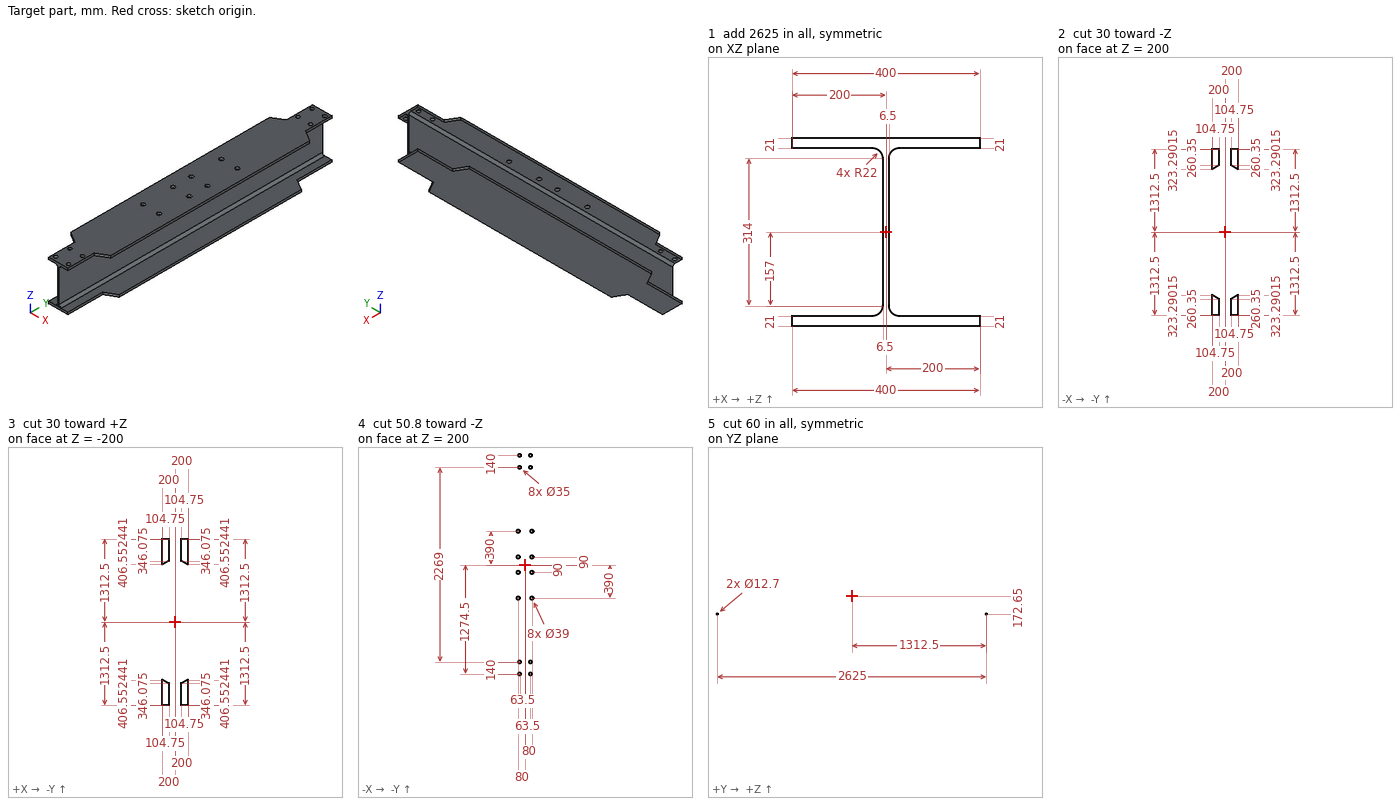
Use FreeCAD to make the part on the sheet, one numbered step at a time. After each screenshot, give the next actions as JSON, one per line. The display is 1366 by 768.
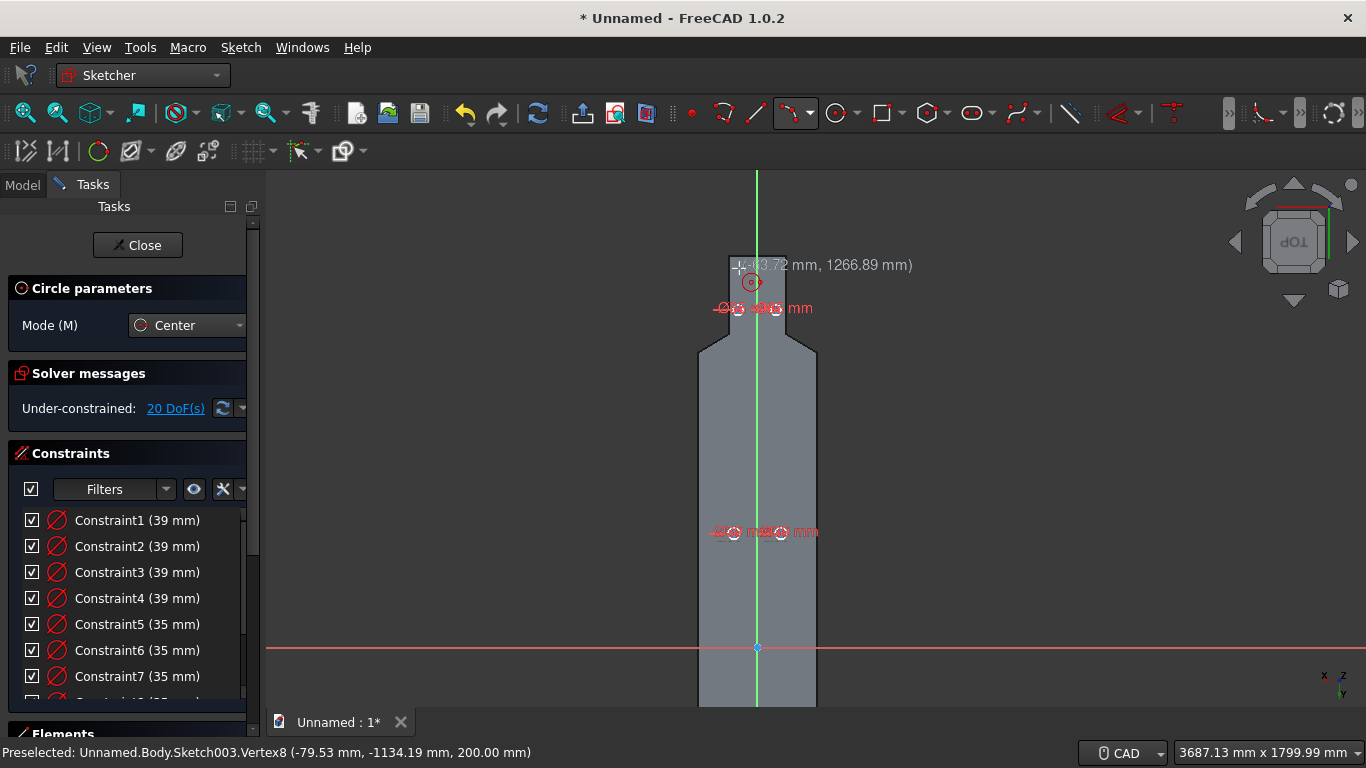
{"action": "left_click", "coordinate": [739, 268]}
{"action": "mouse_move", "coordinate": [742, 264]}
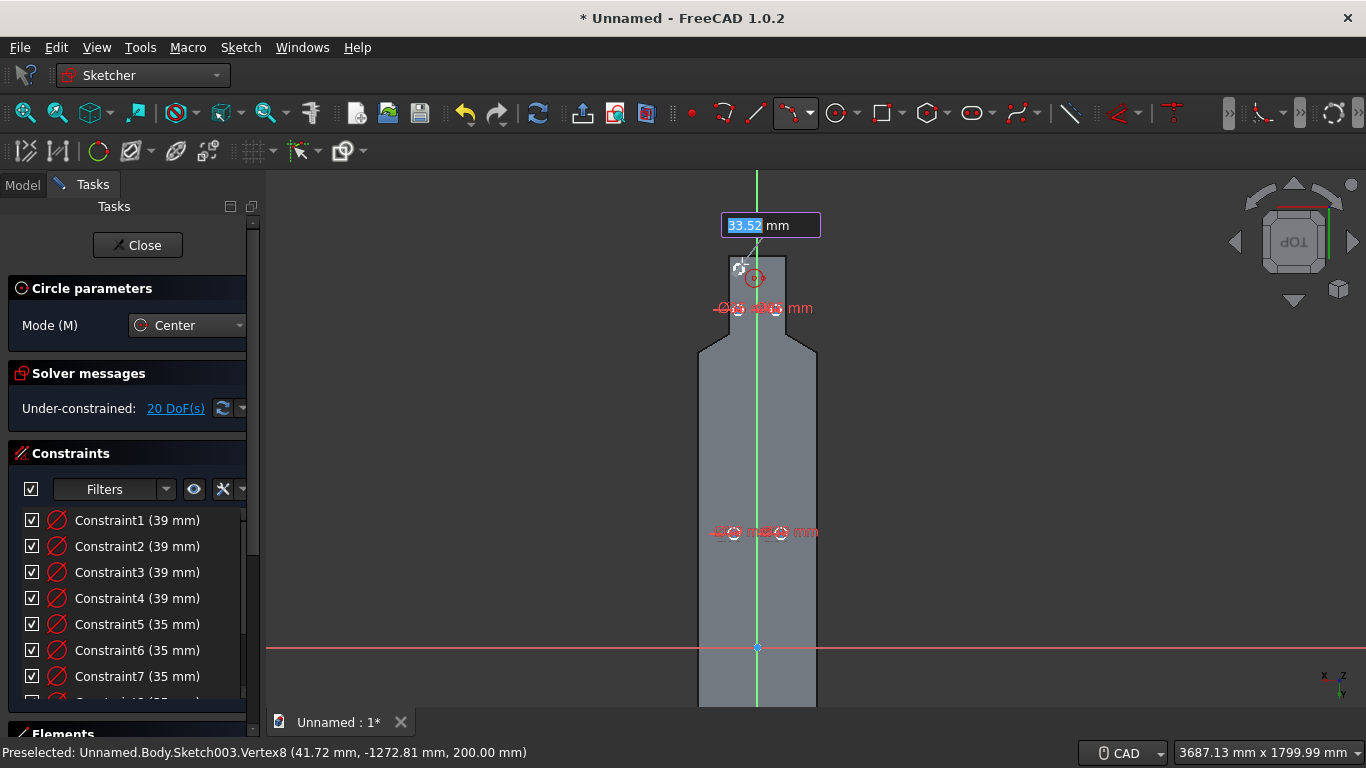
{"action": "type", "text": "35"}
{"action": "key", "text": "Return"}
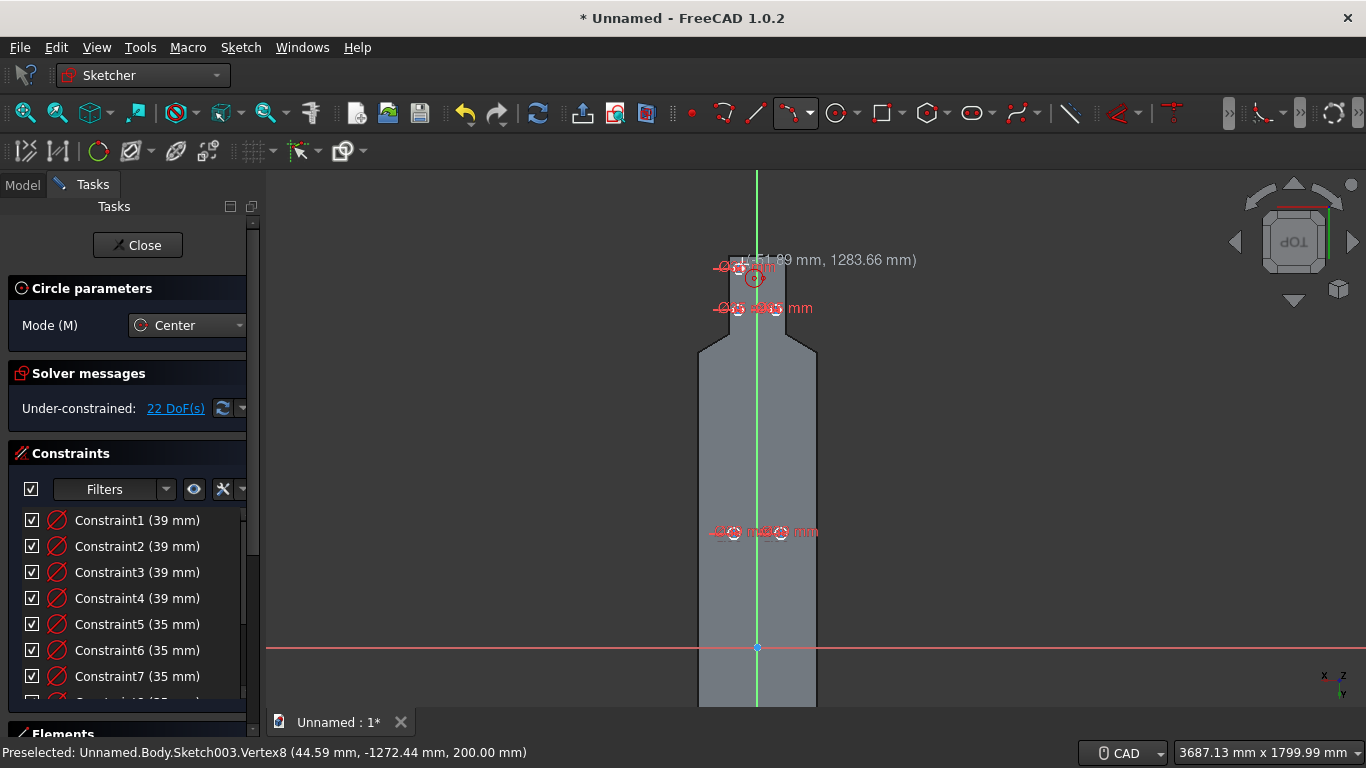
{"action": "scroll", "coordinate": [776, 268], "scroll_direction": "up", "scroll_amount": 8}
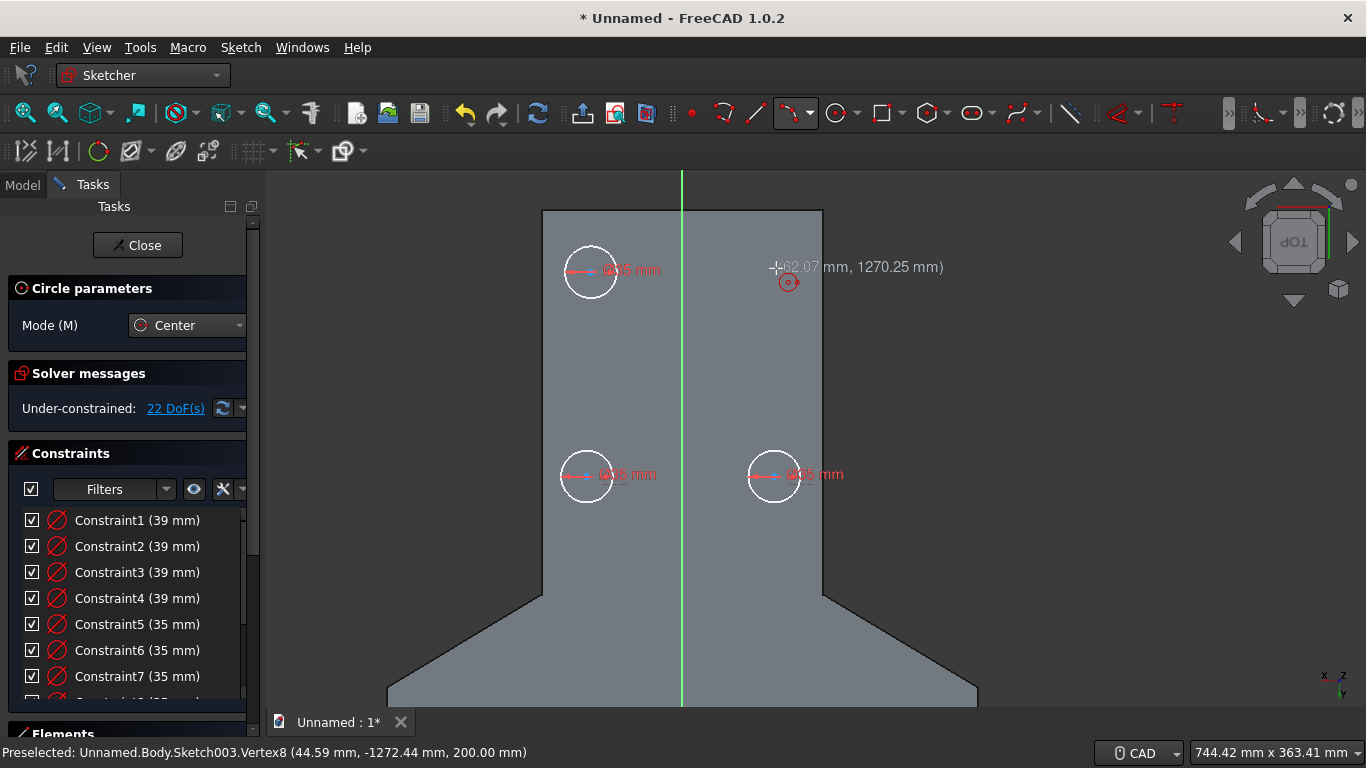
{"action": "scroll", "coordinate": [754, 268], "scroll_direction": "down", "scroll_amount": 12}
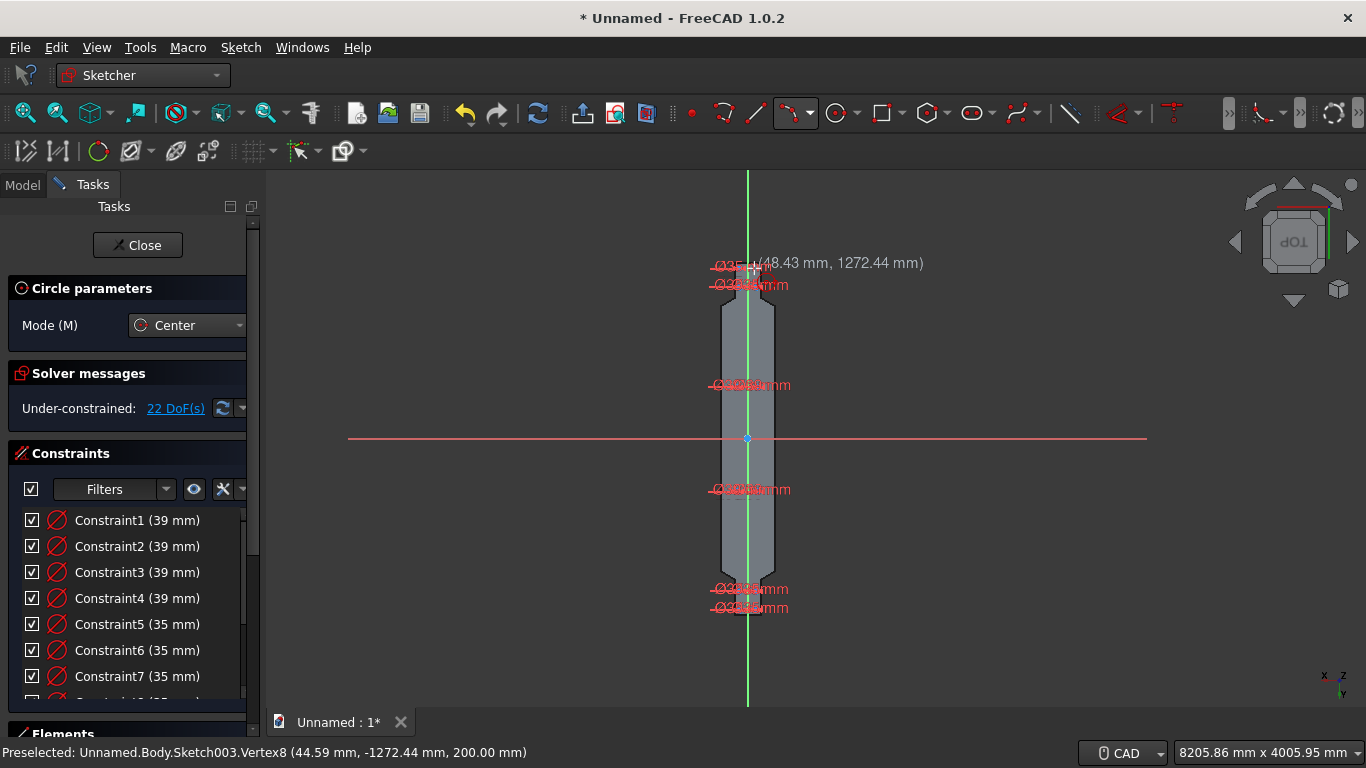
{"action": "scroll", "coordinate": [756, 268], "scroll_direction": "up", "scroll_amount": 4}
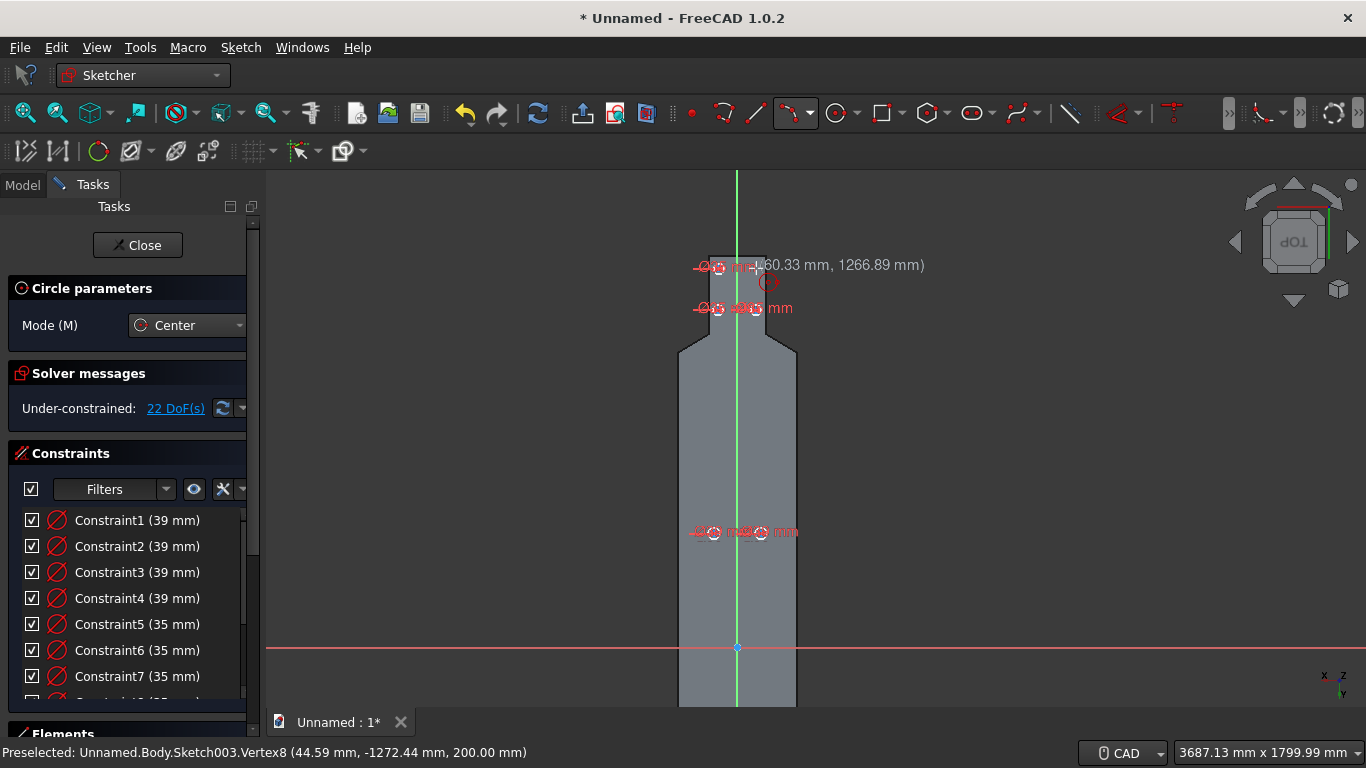
{"action": "left_click", "coordinate": [756, 268]}
{"action": "mouse_move", "coordinate": [760, 264]}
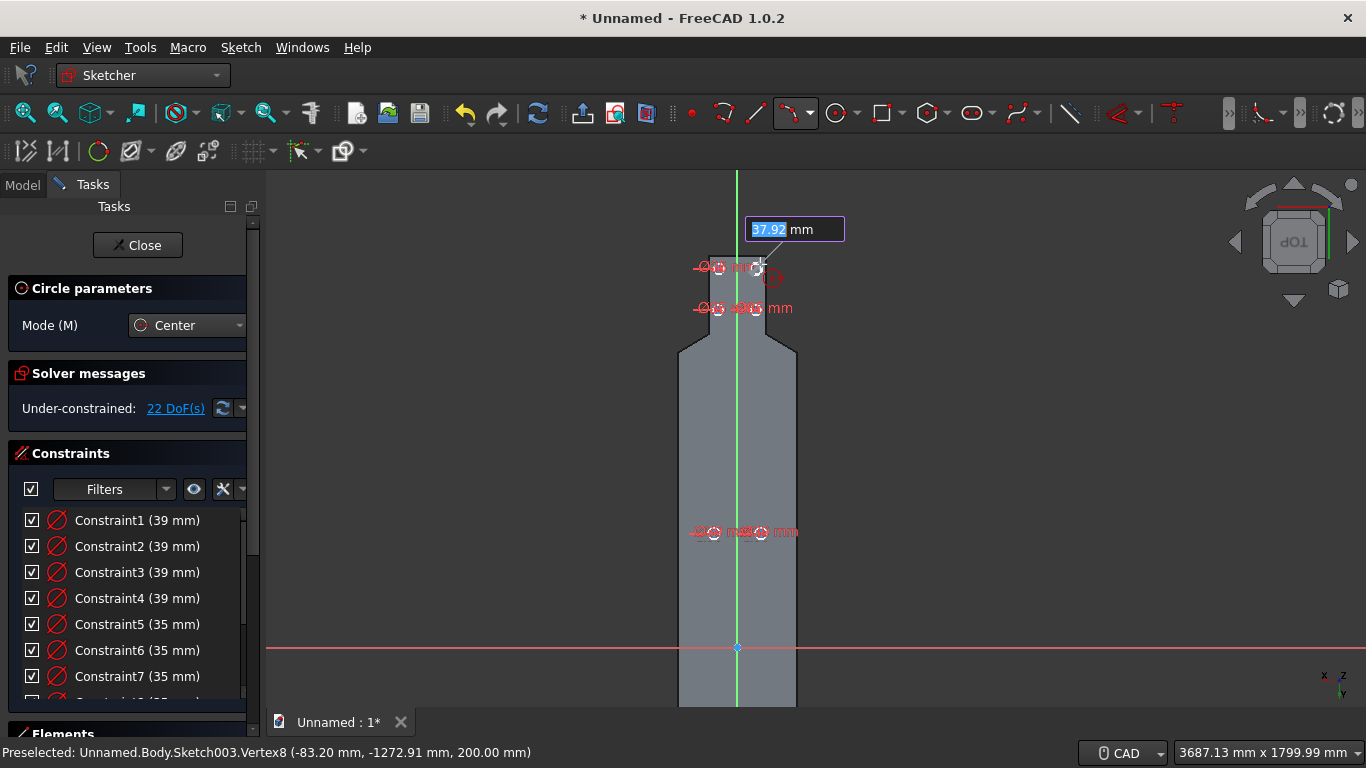
{"action": "type", "text": "35"}
{"action": "key", "text": "Return"}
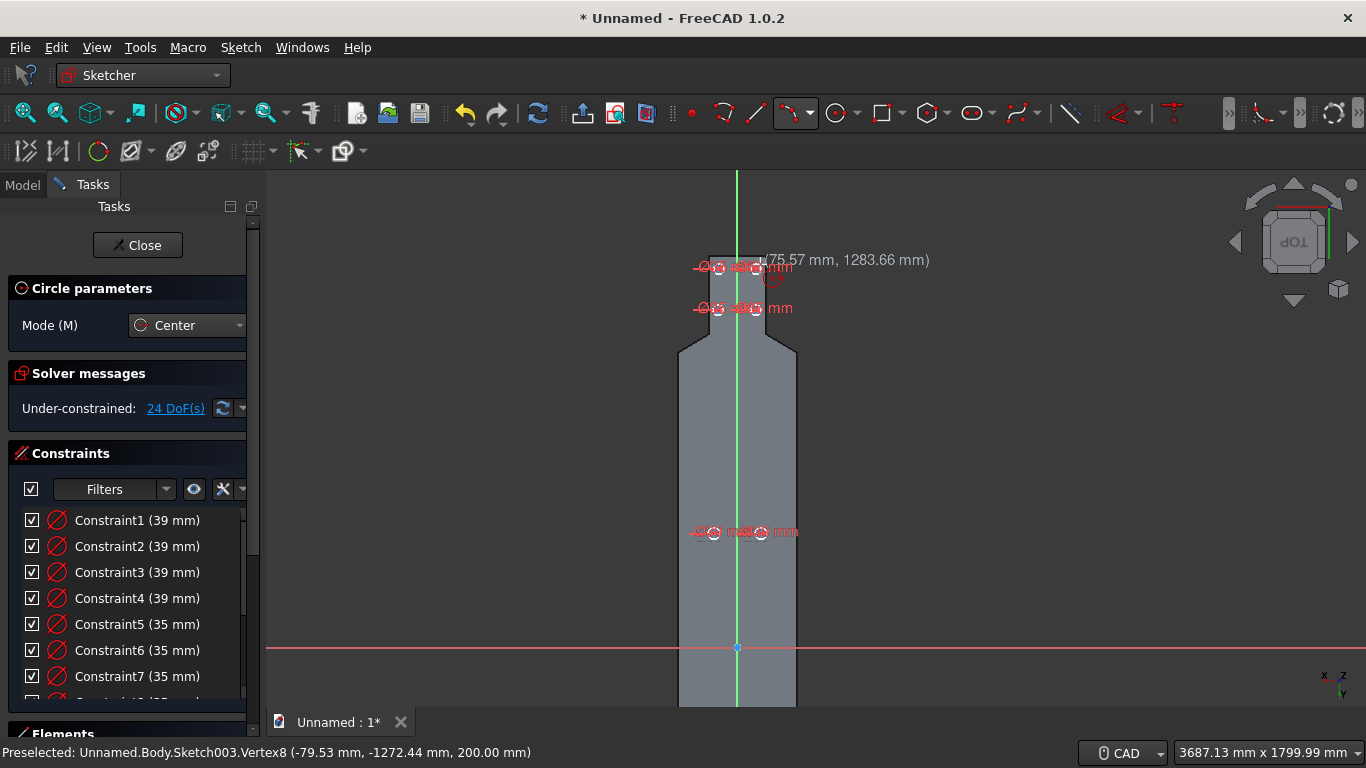
{"action": "scroll", "coordinate": [761, 675], "scroll_direction": "up", "scroll_amount": 7}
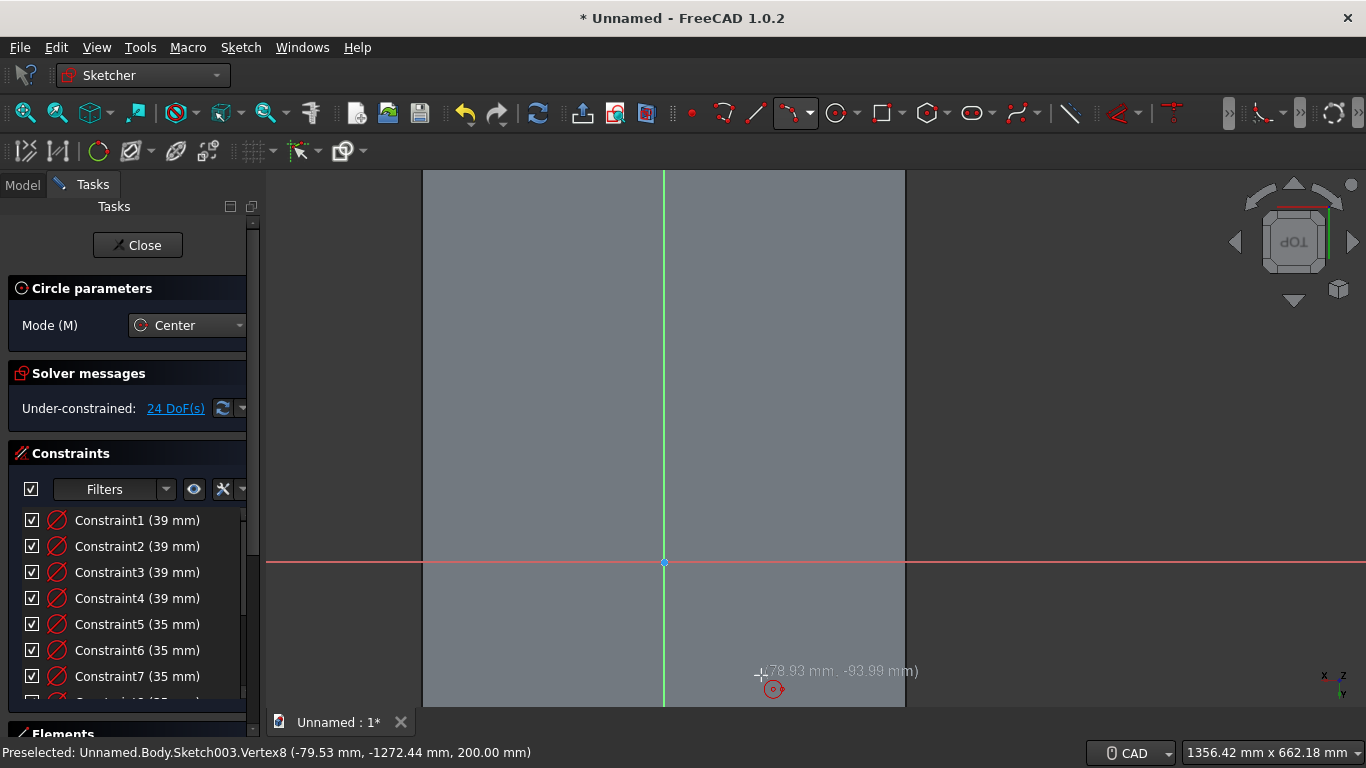
{"action": "scroll", "coordinate": [758, 423], "scroll_direction": "down", "scroll_amount": 11}